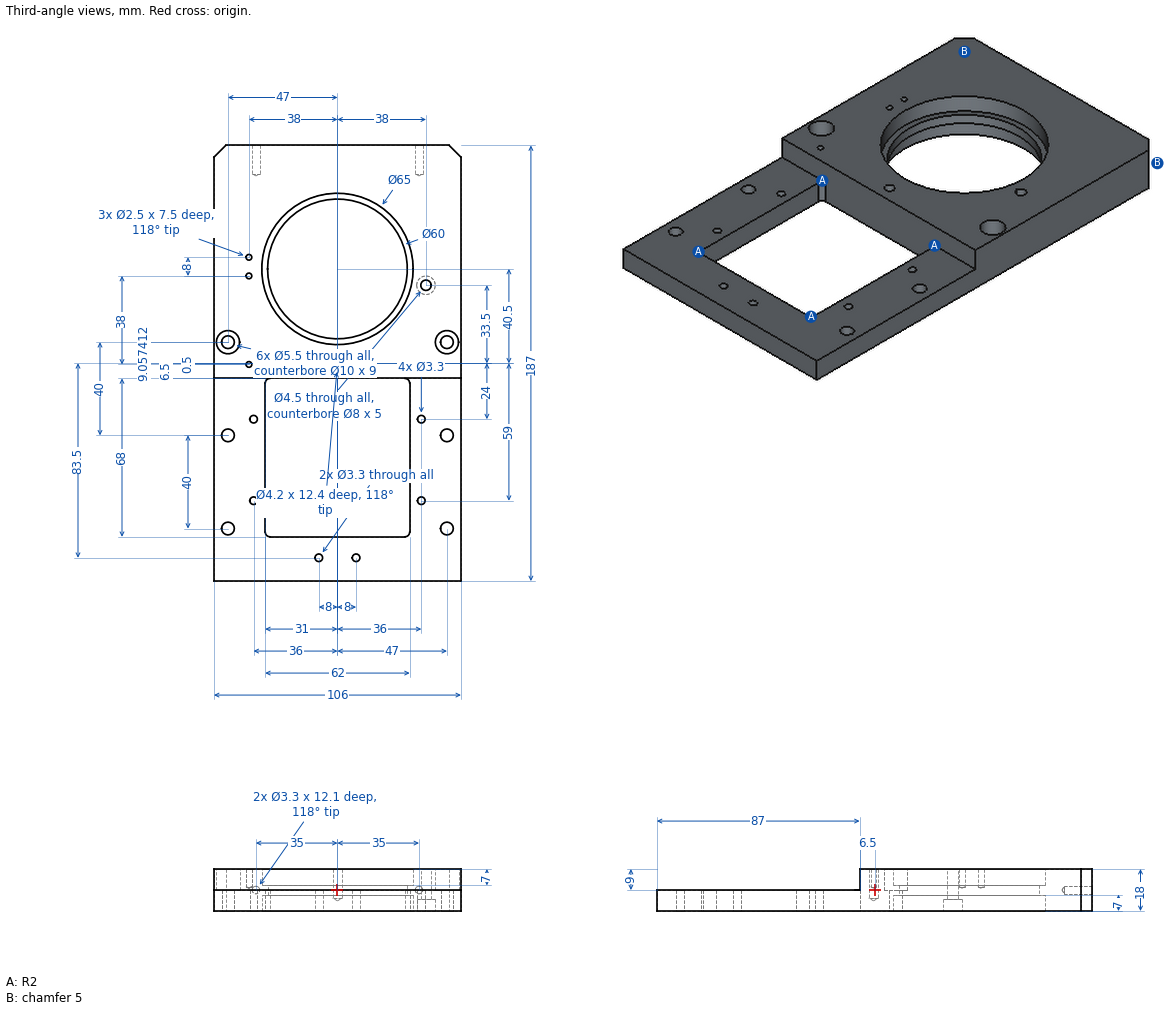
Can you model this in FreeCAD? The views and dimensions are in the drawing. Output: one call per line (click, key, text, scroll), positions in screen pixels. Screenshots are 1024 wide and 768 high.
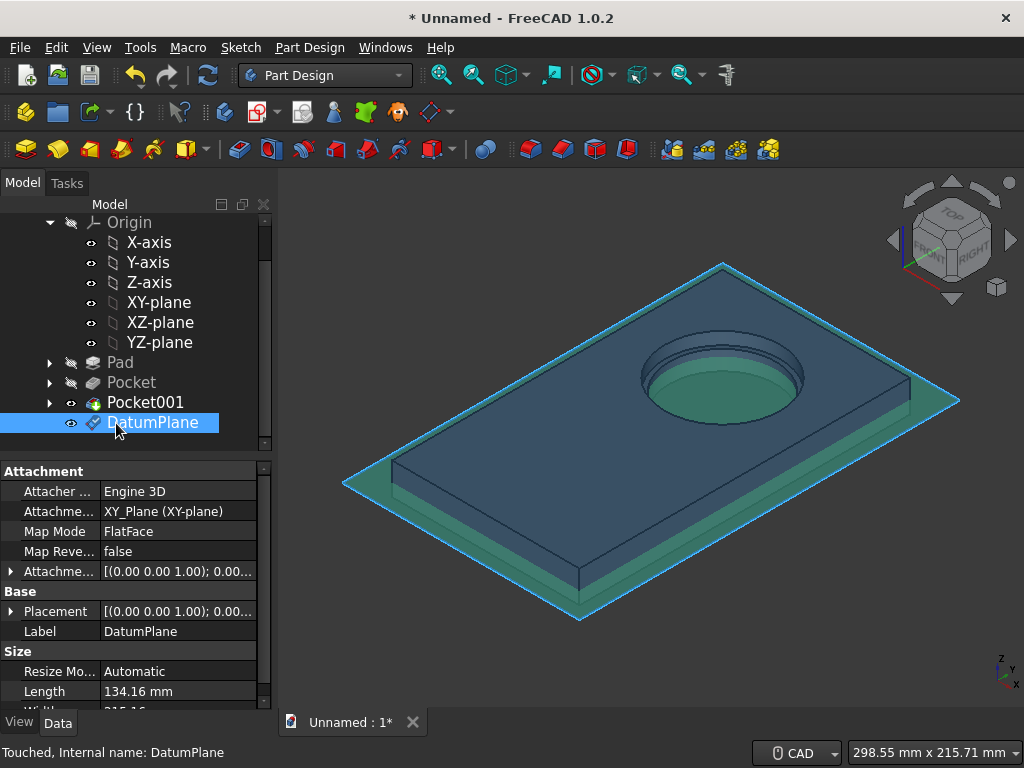
click(258, 112)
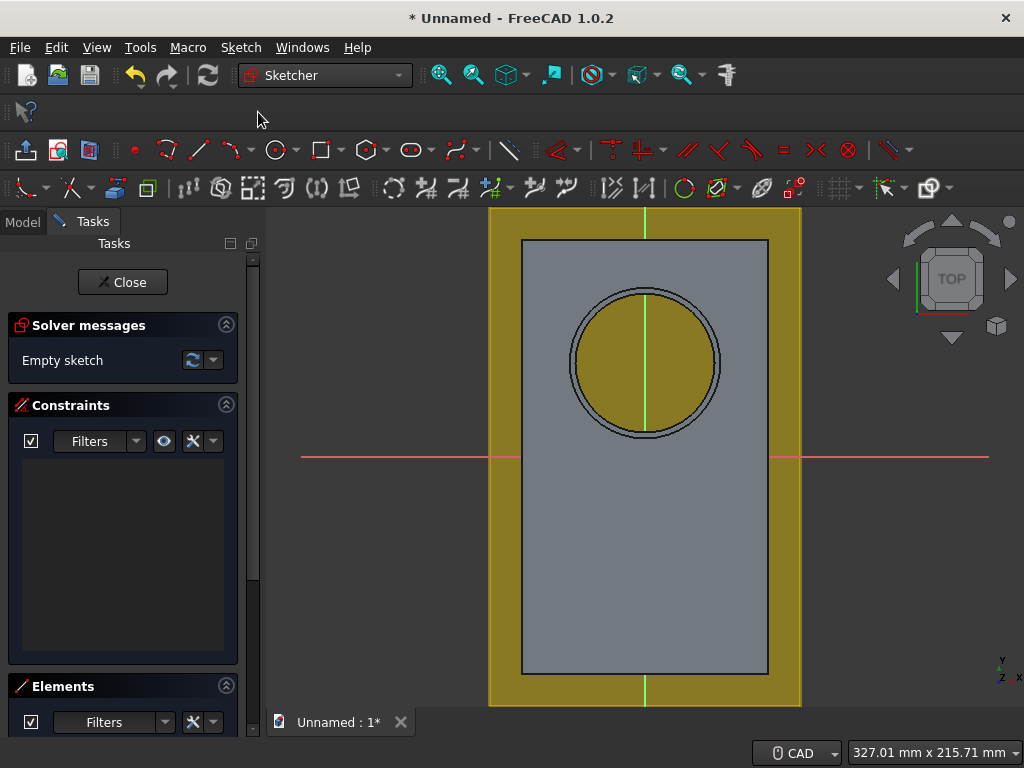
click(90, 150)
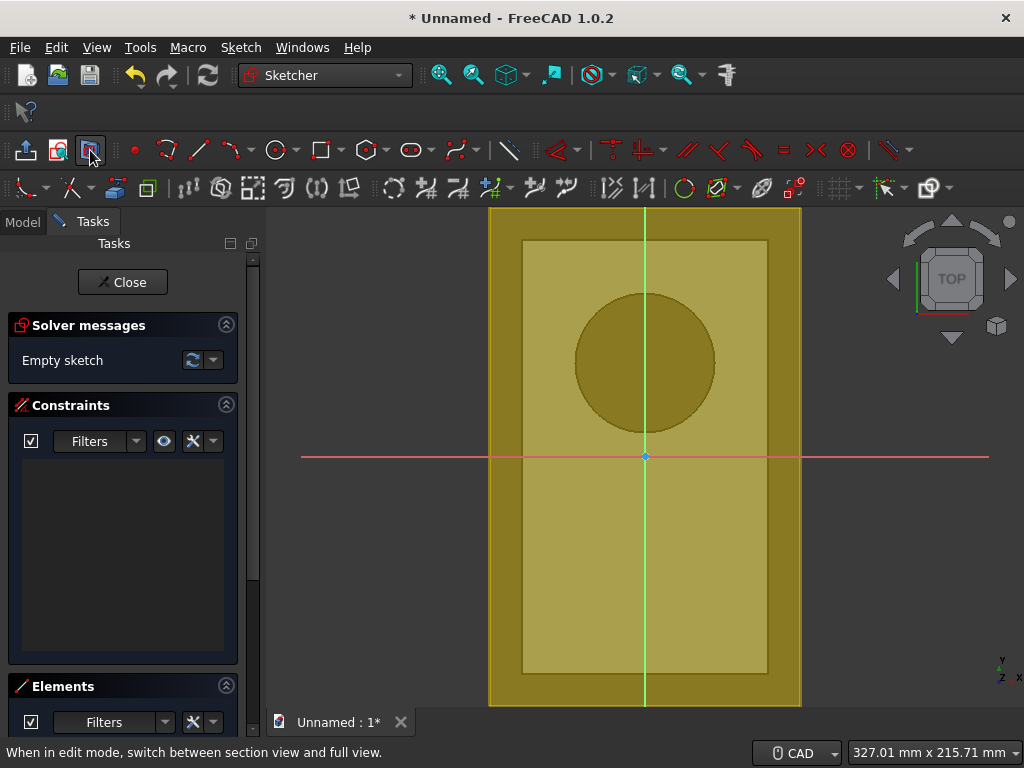
scroll(728, 269, up, 3)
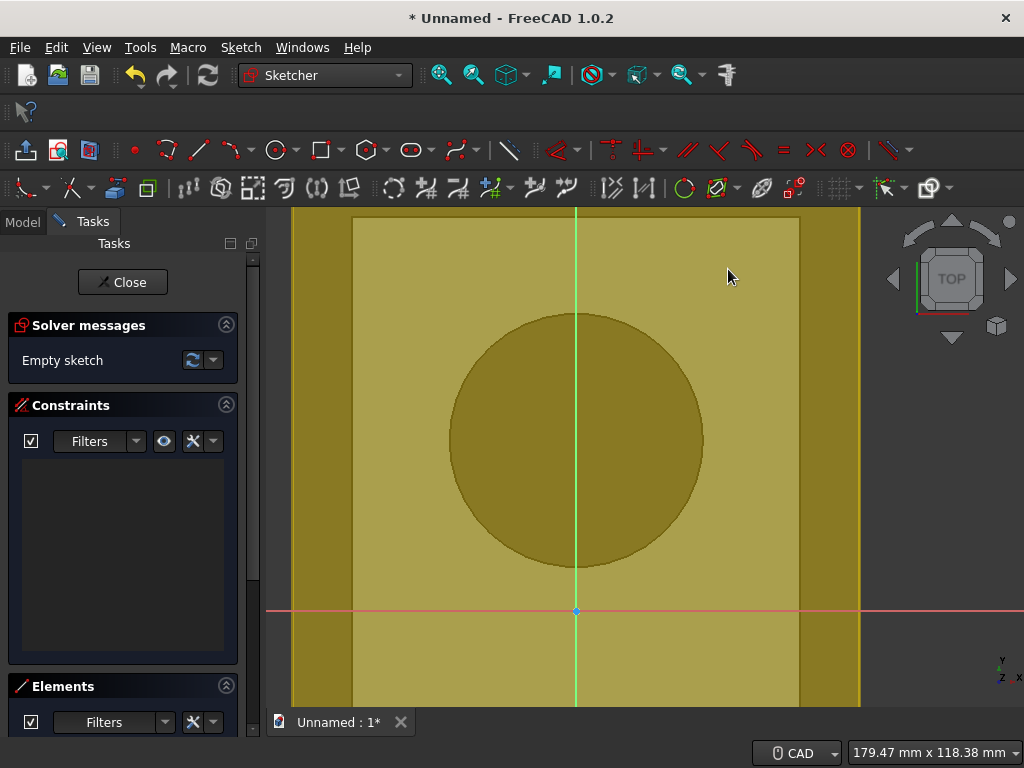
click(276, 150)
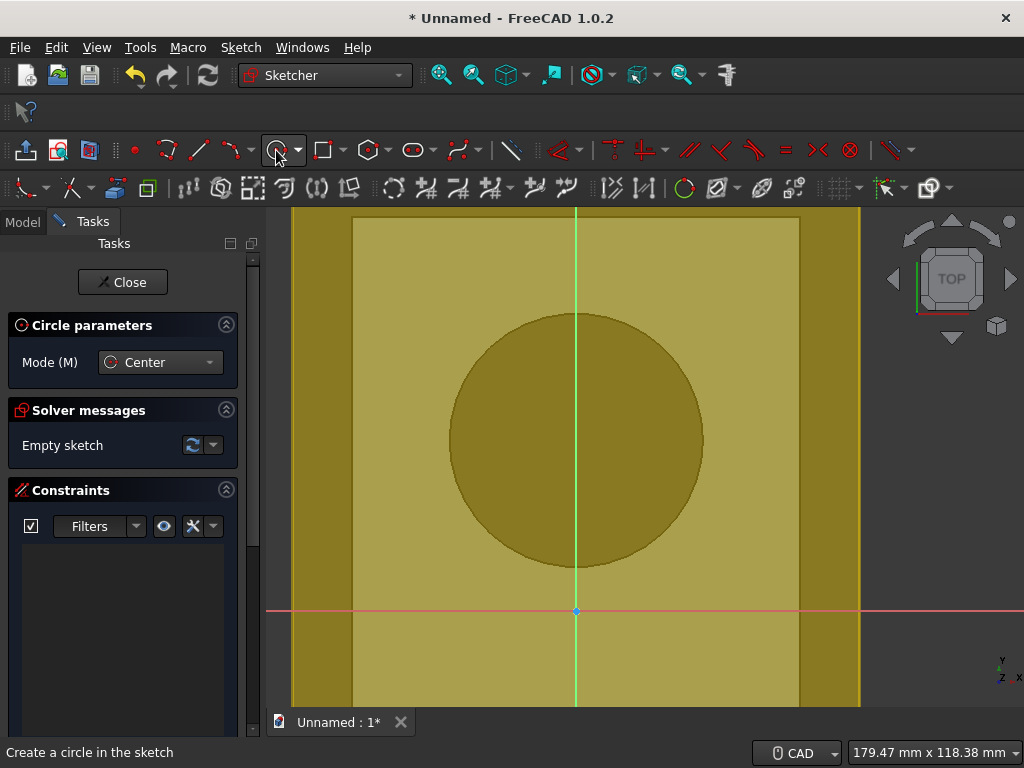
click(576, 440)
click(673, 343)
key(Escape)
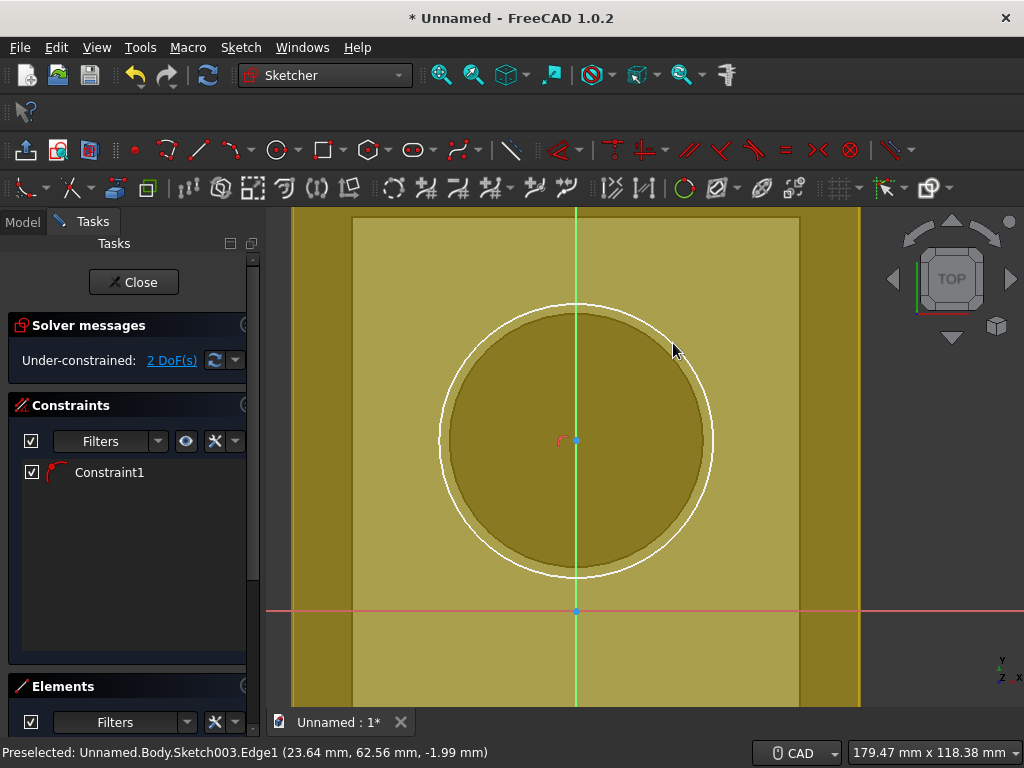
click(558, 150)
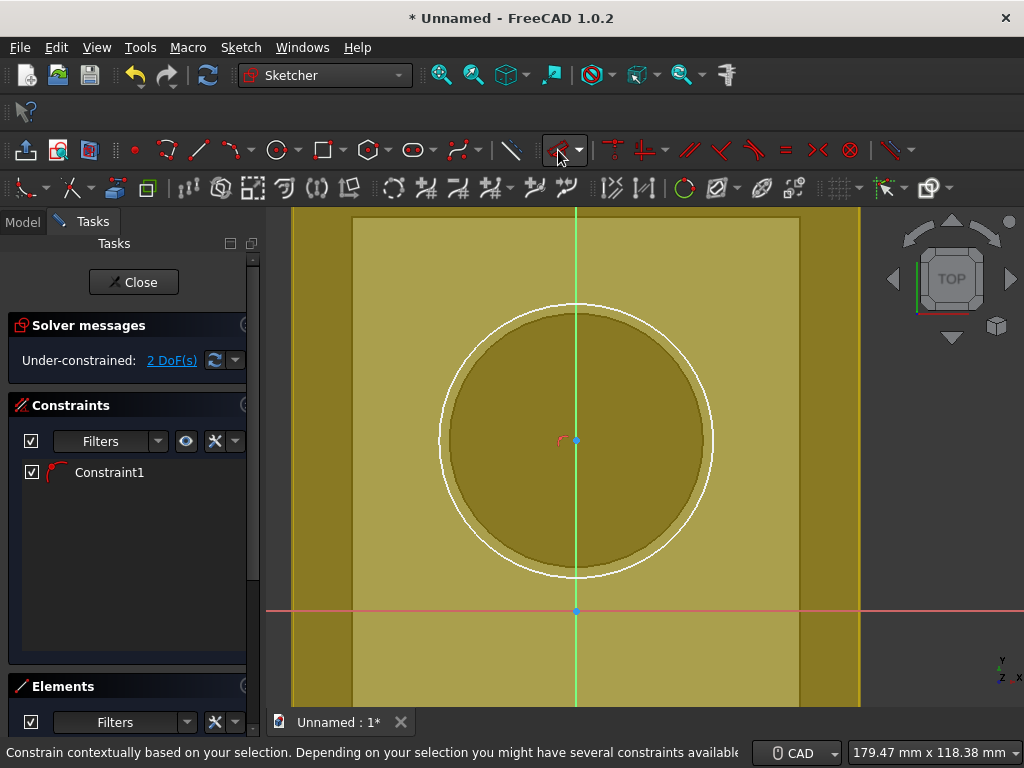
click(673, 344)
click(696, 321)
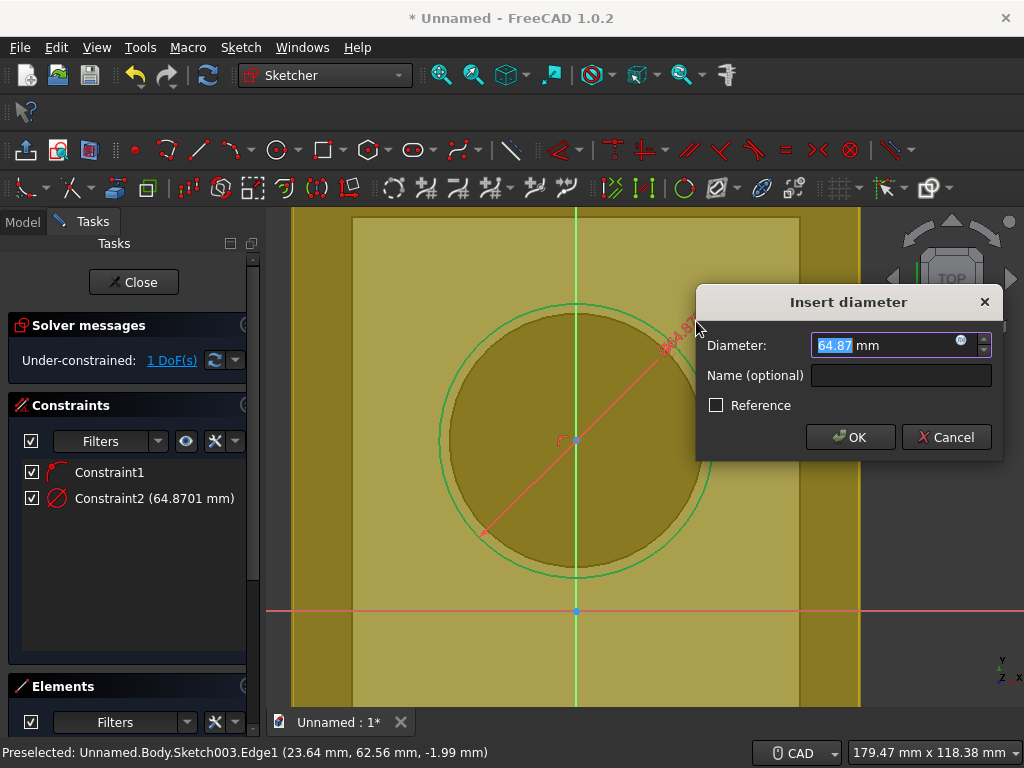
text(65)
key(Return)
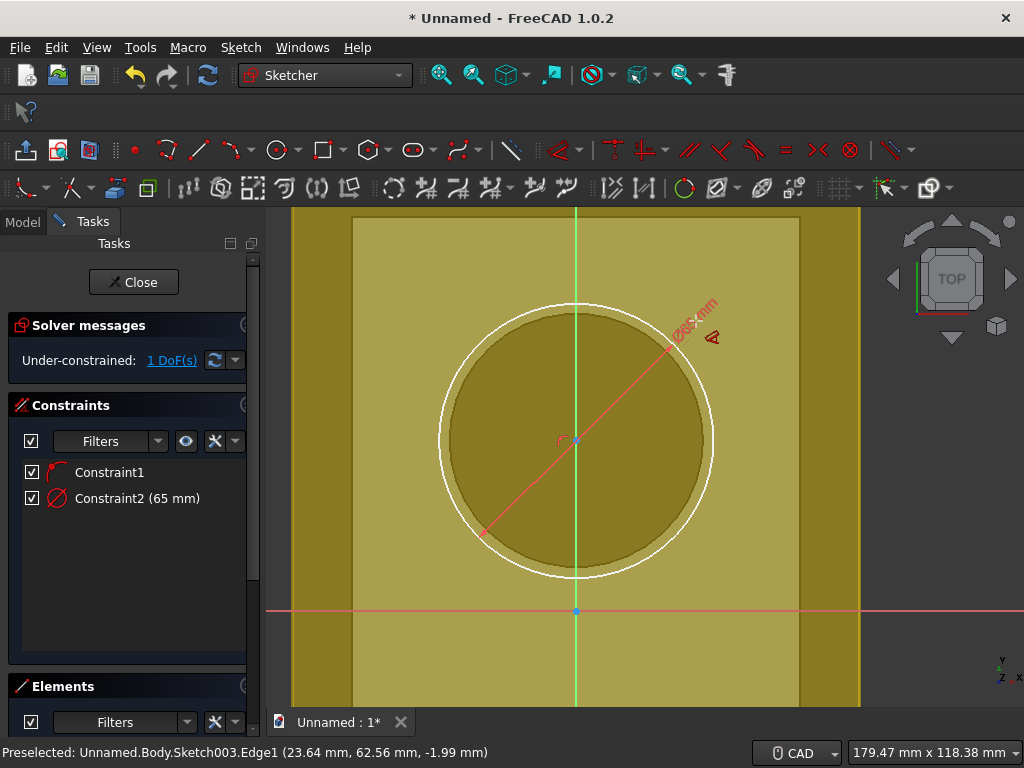
click(576, 441)
click(610, 526)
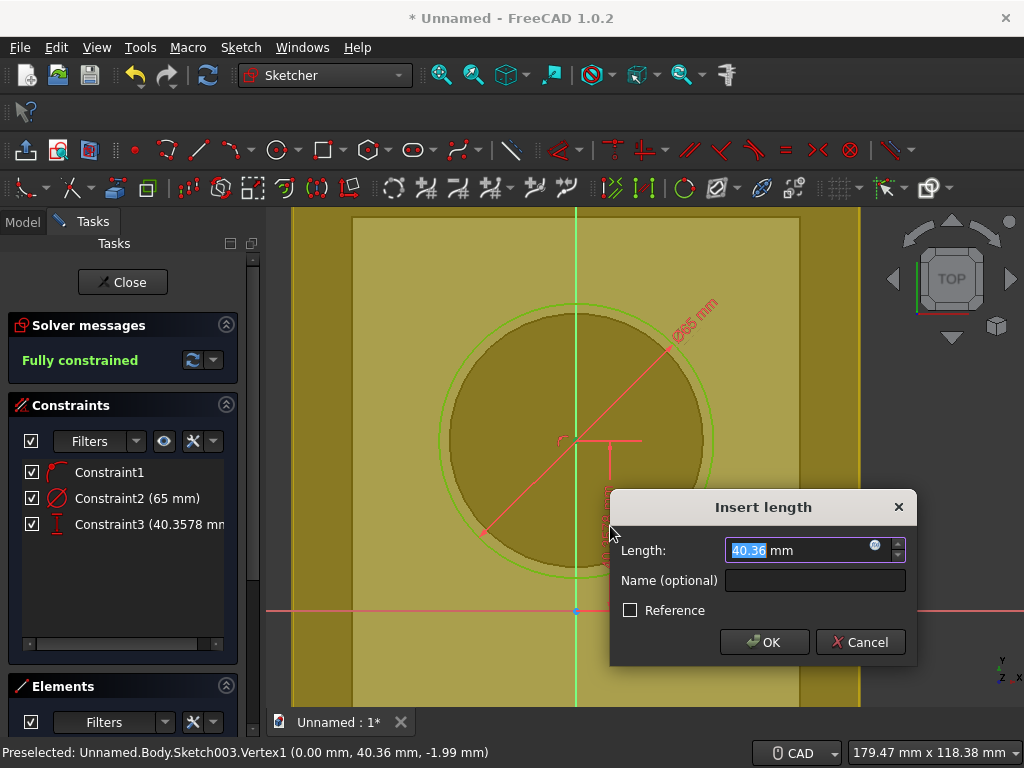
text(40.5)
key(Return)
key(Escape)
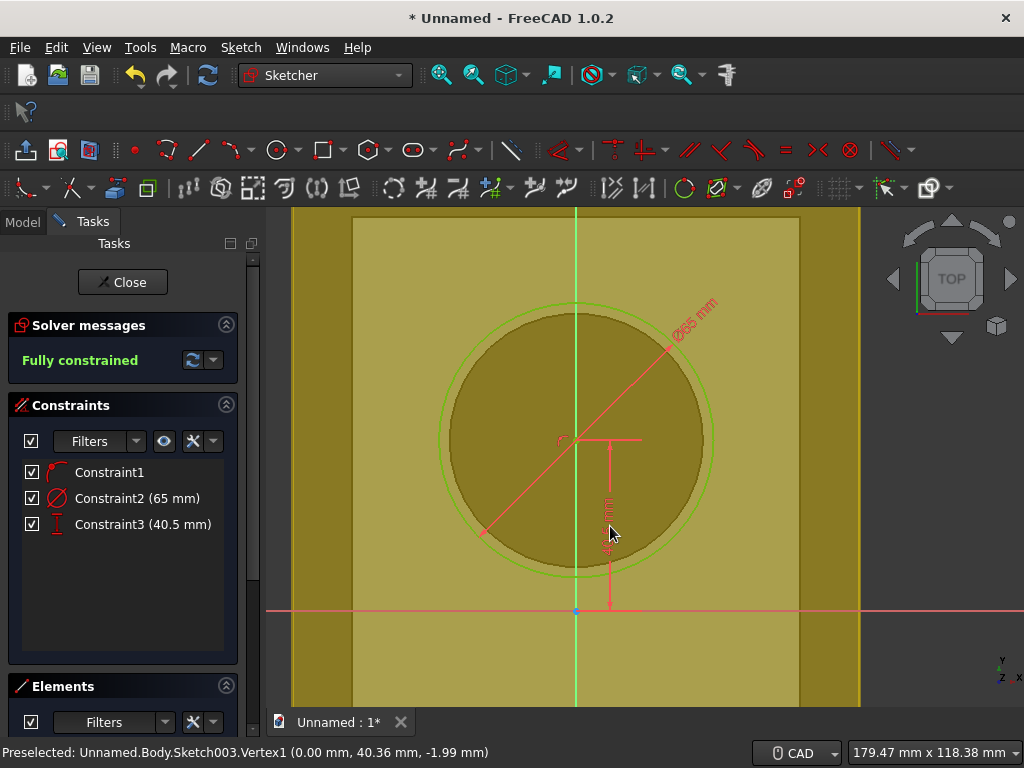
click(123, 282)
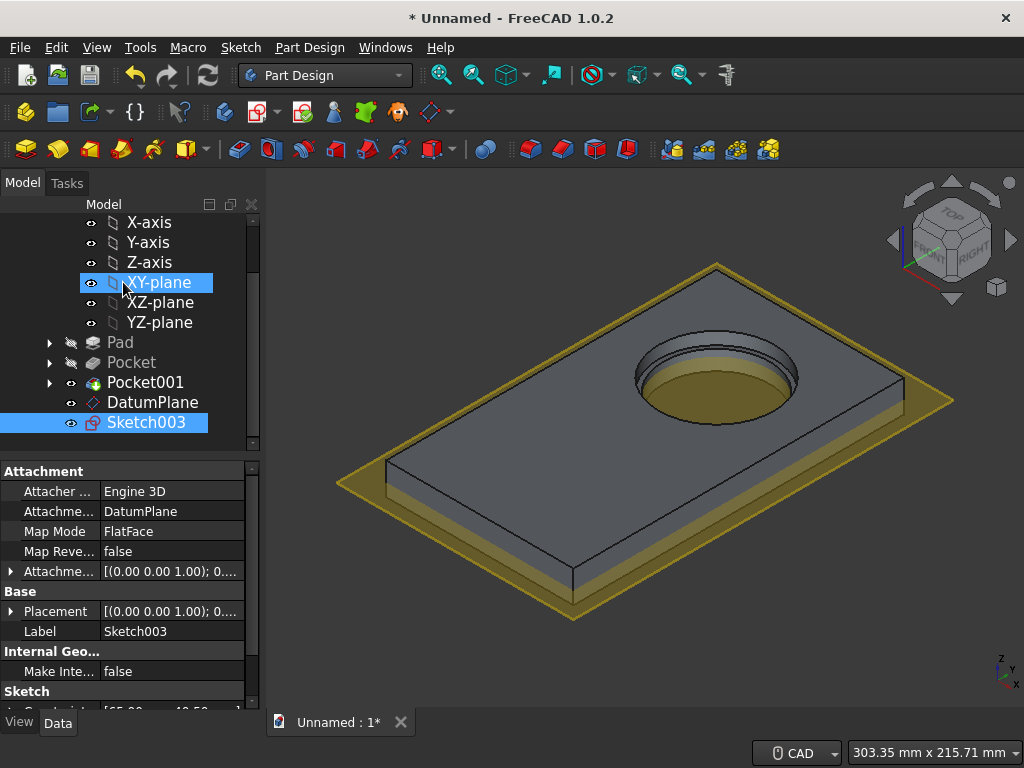
click(240, 150)